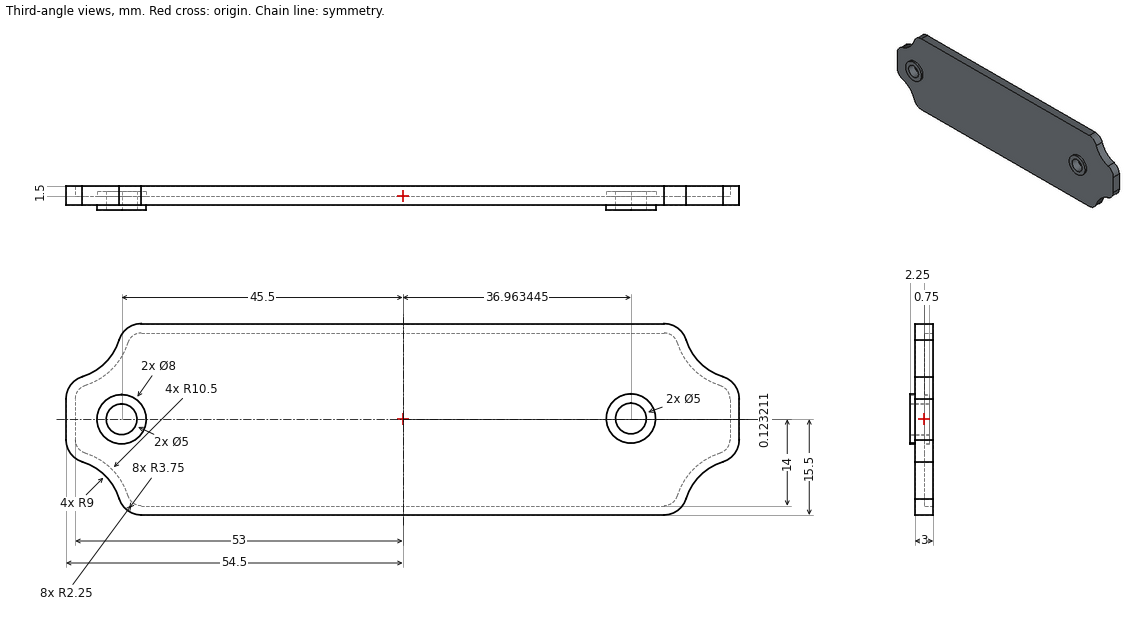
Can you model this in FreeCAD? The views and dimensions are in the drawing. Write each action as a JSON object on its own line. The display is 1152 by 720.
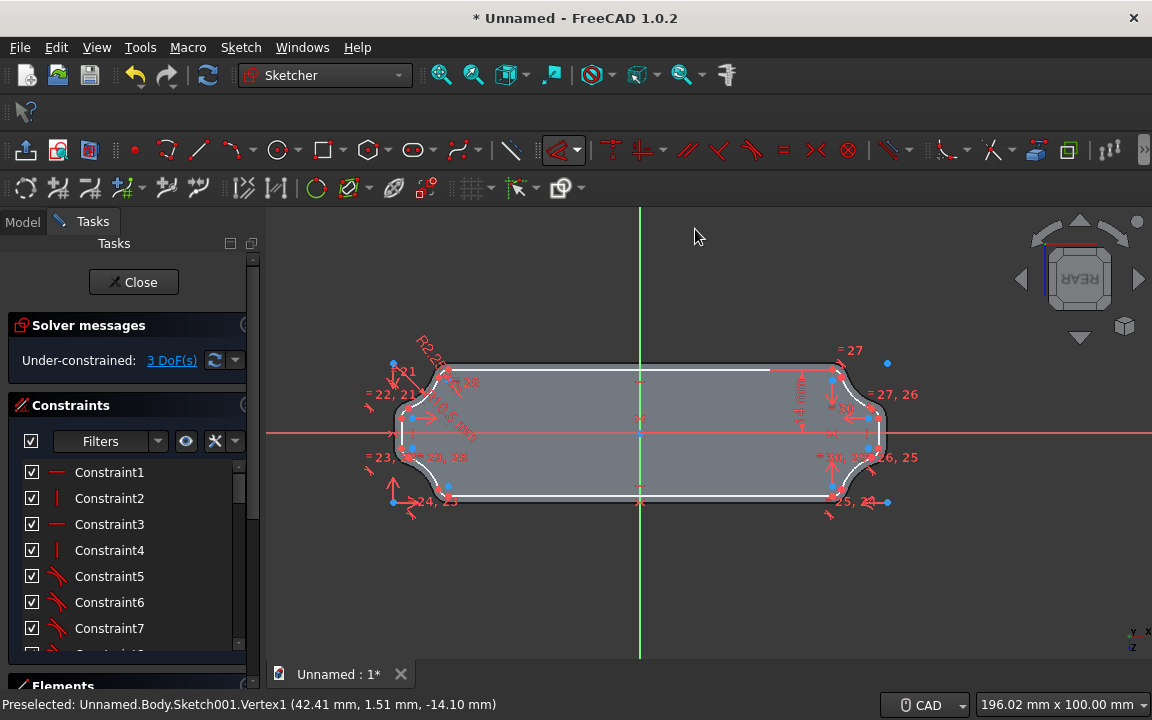
{"action": "left_click", "coordinate": [402, 418]}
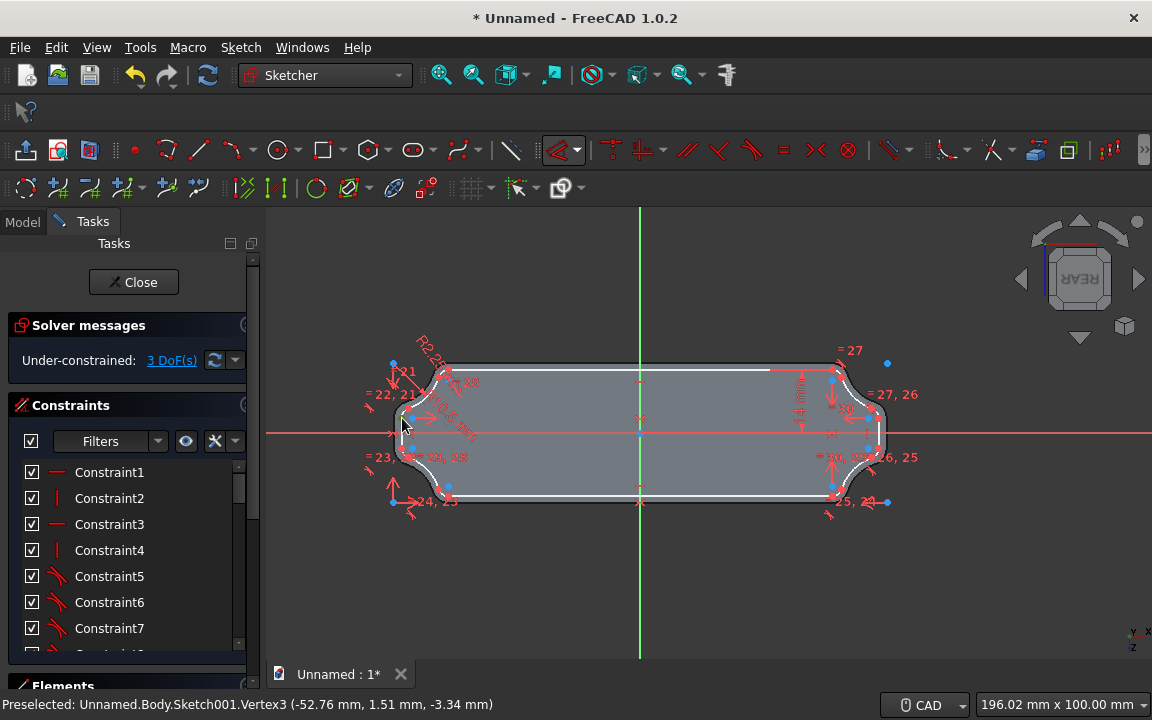
{"action": "key", "text": "l"}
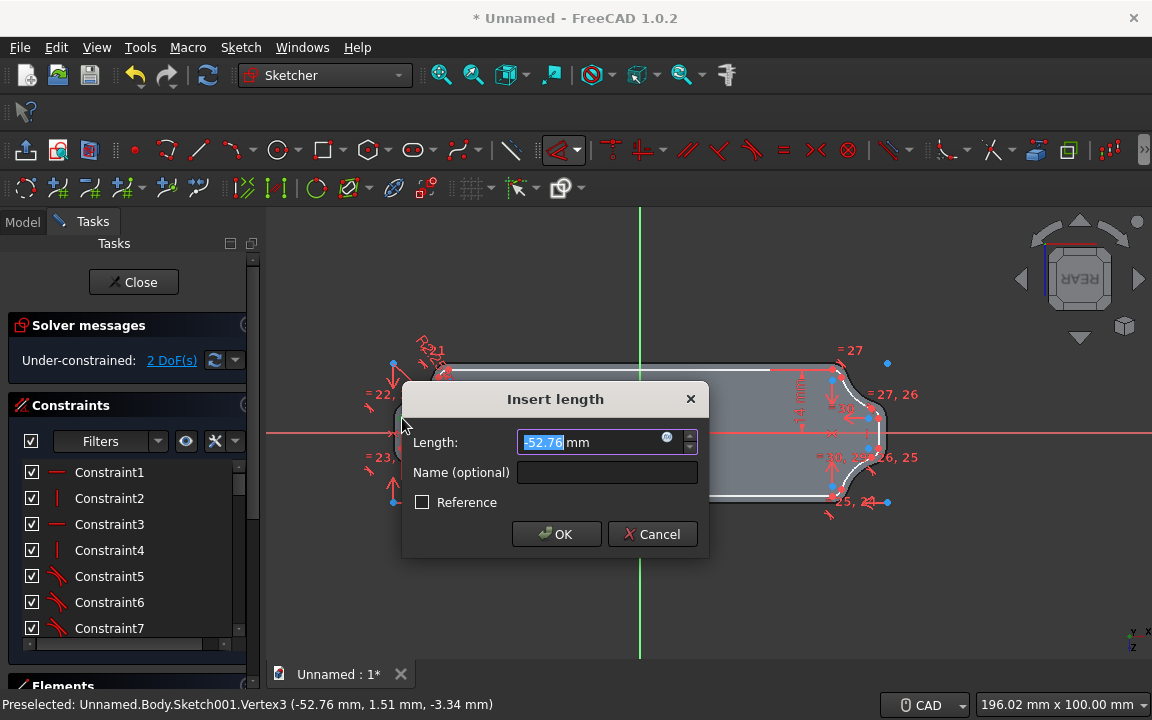
{"action": "type", "text": "-53"}
{"action": "key", "text": "Return"}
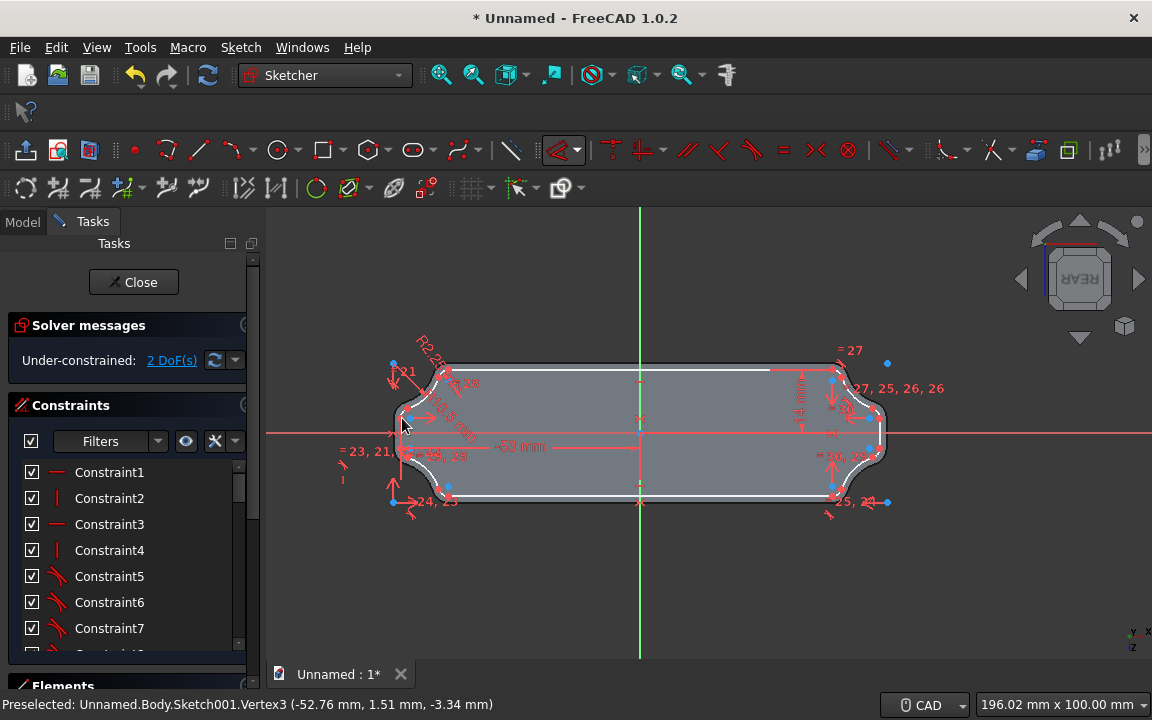
{"action": "left_click", "coordinate": [393, 363]}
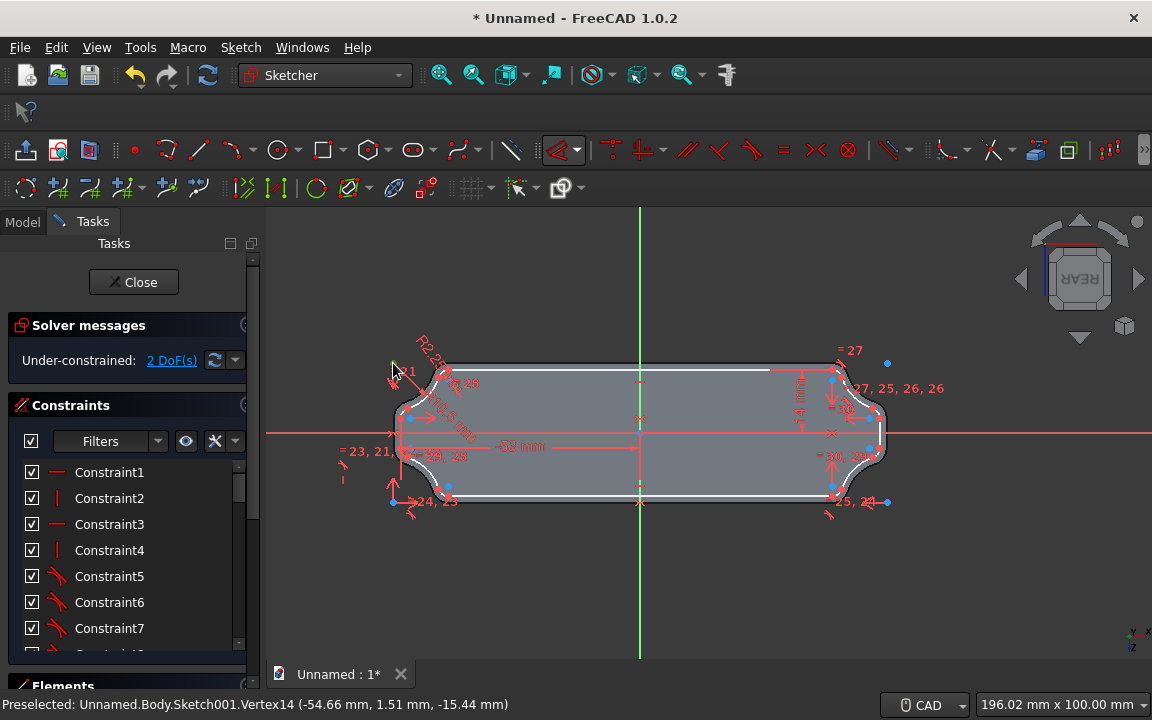
{"action": "left_click", "coordinate": [580, 150]}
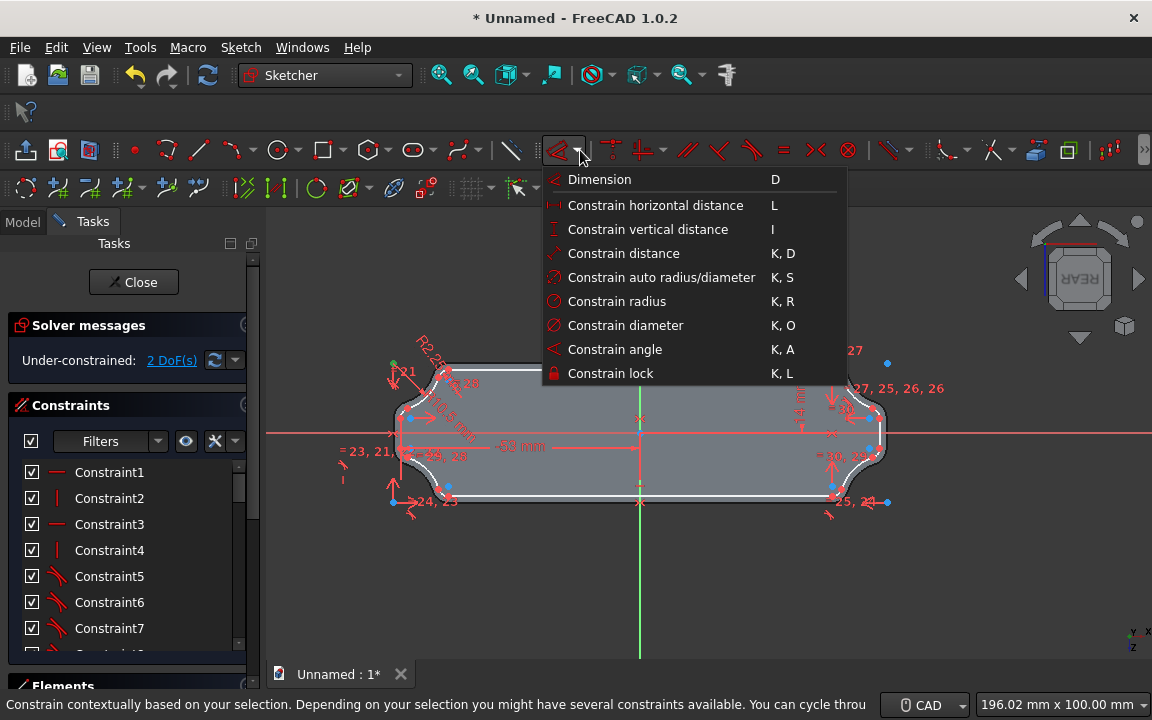
{"action": "left_click", "coordinate": [695, 205]}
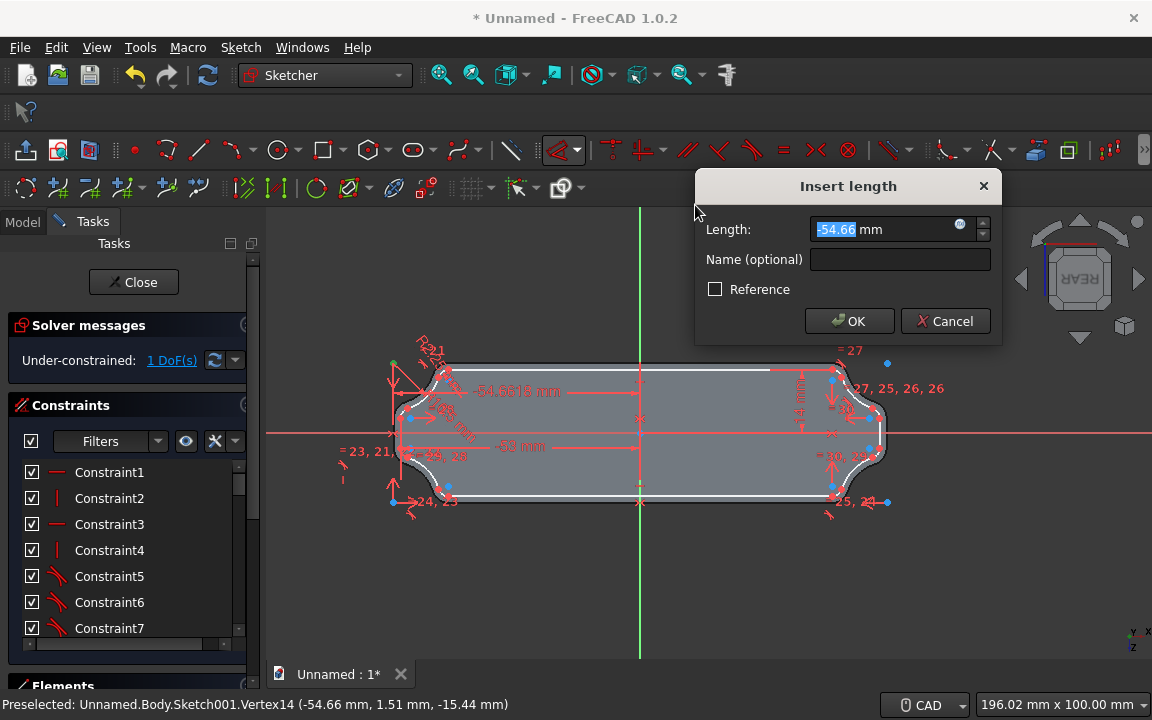
{"action": "type", "text": "-54.5"}
{"action": "key", "text": "Return"}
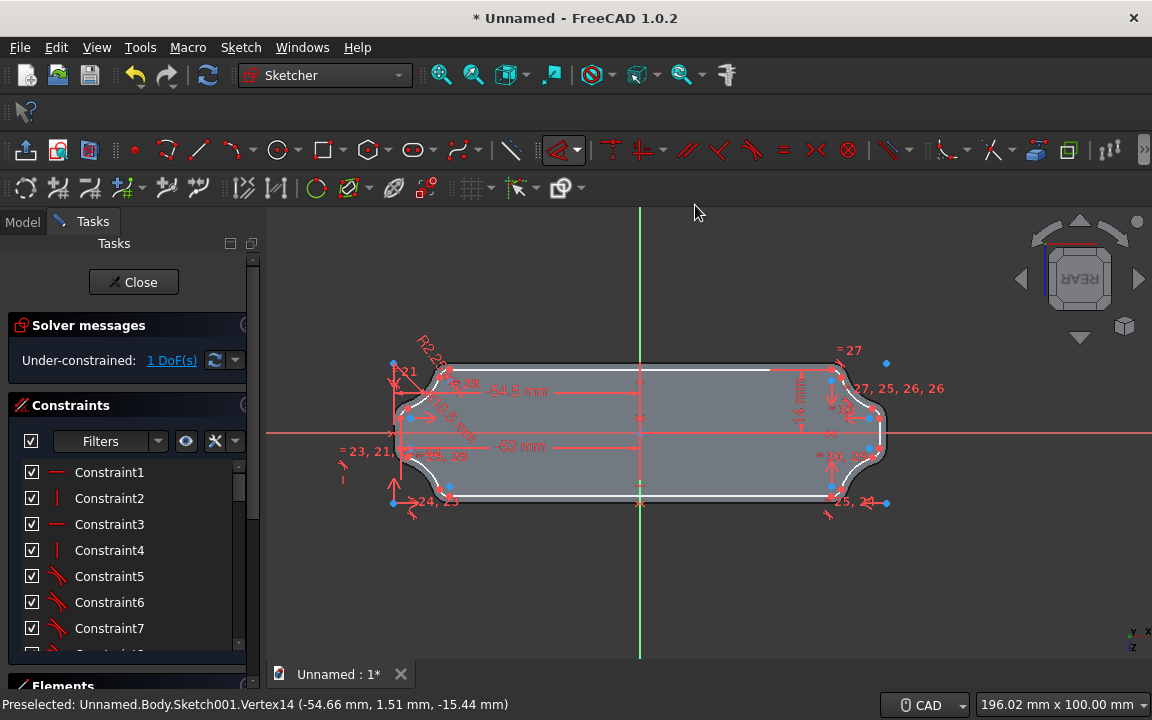
{"action": "left_click", "coordinate": [394, 363]}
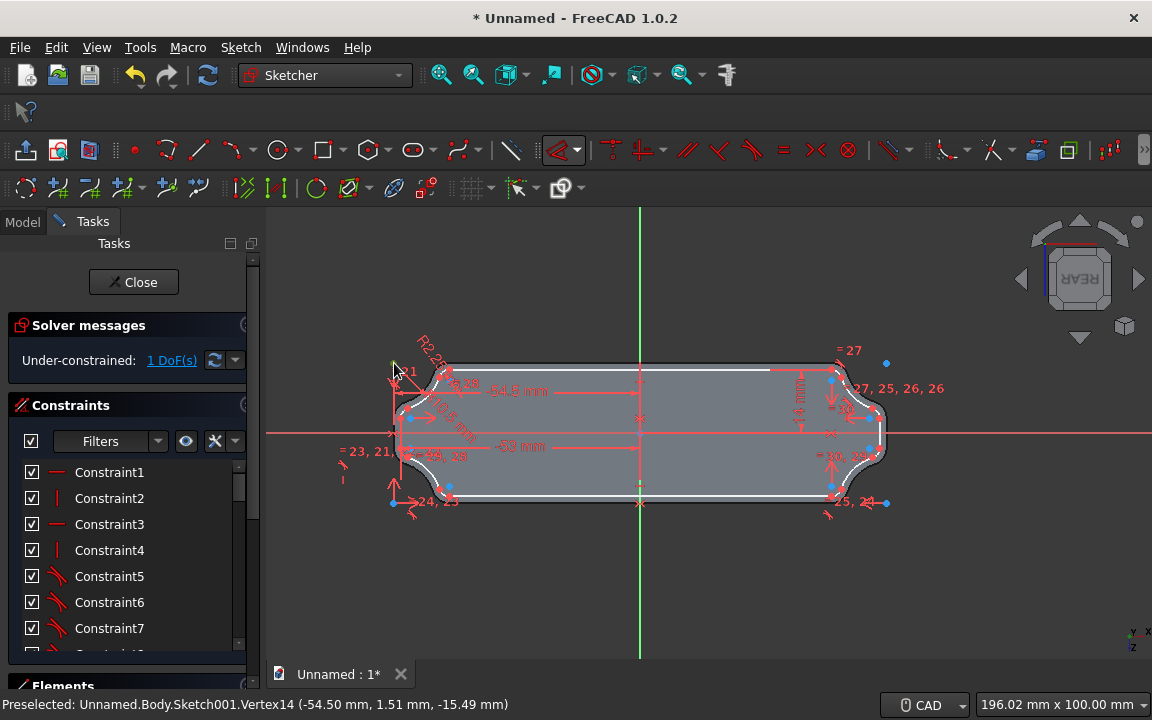
{"action": "key", "text": "i"}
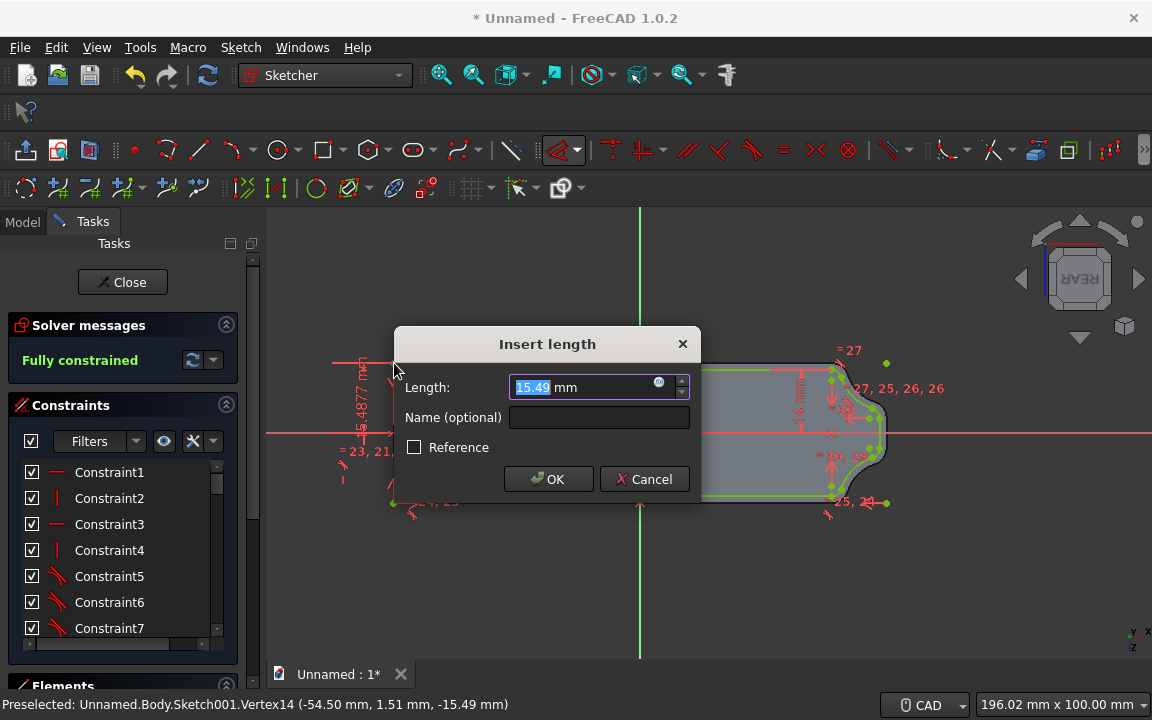
{"action": "type", "text": "15.5"}
{"action": "key", "text": "Return"}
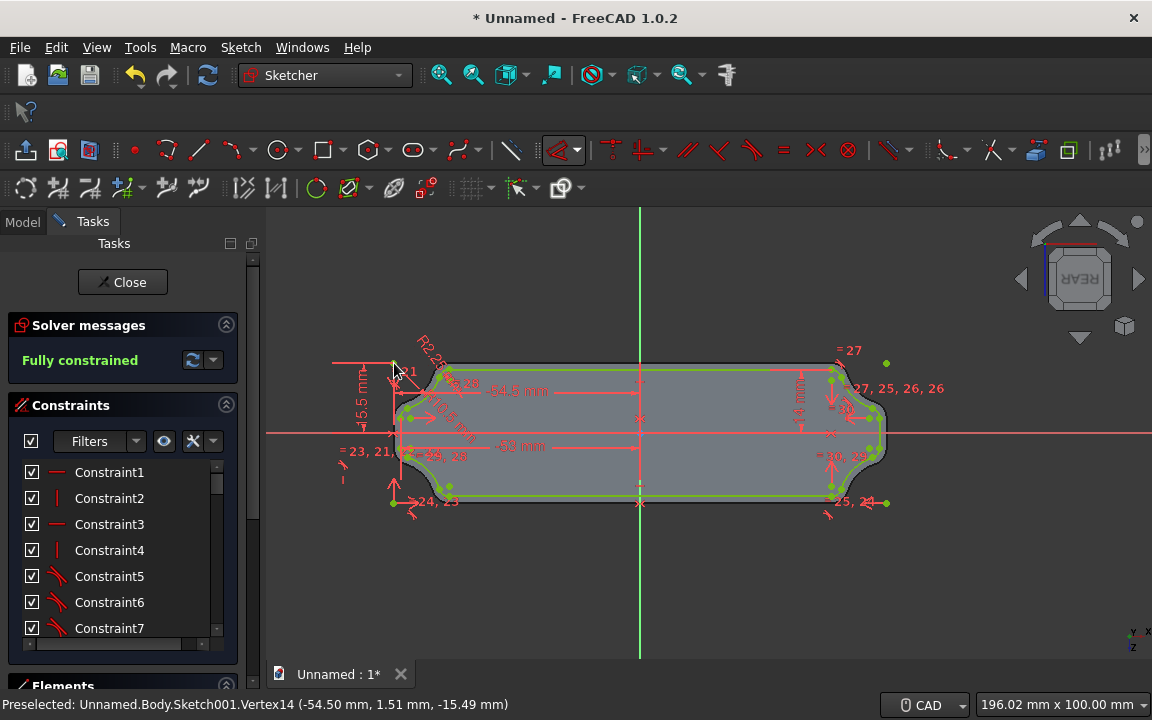
{"action": "left_click", "coordinate": [123, 282]}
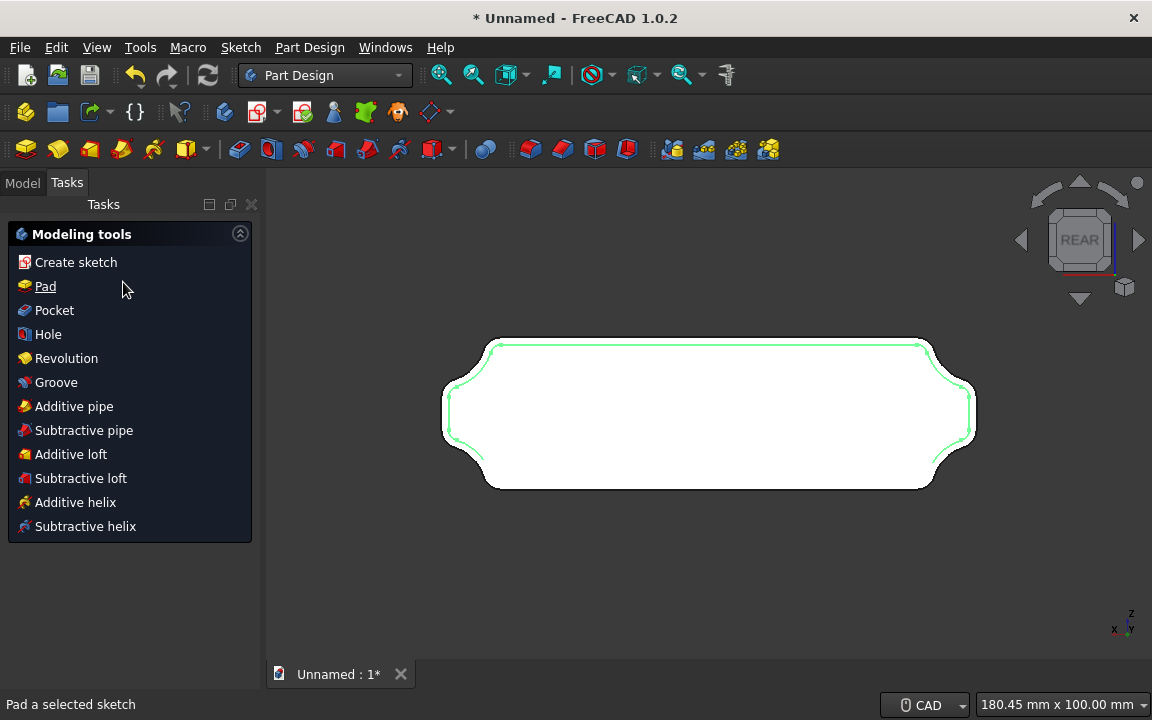
{"action": "left_click", "coordinate": [240, 150]}